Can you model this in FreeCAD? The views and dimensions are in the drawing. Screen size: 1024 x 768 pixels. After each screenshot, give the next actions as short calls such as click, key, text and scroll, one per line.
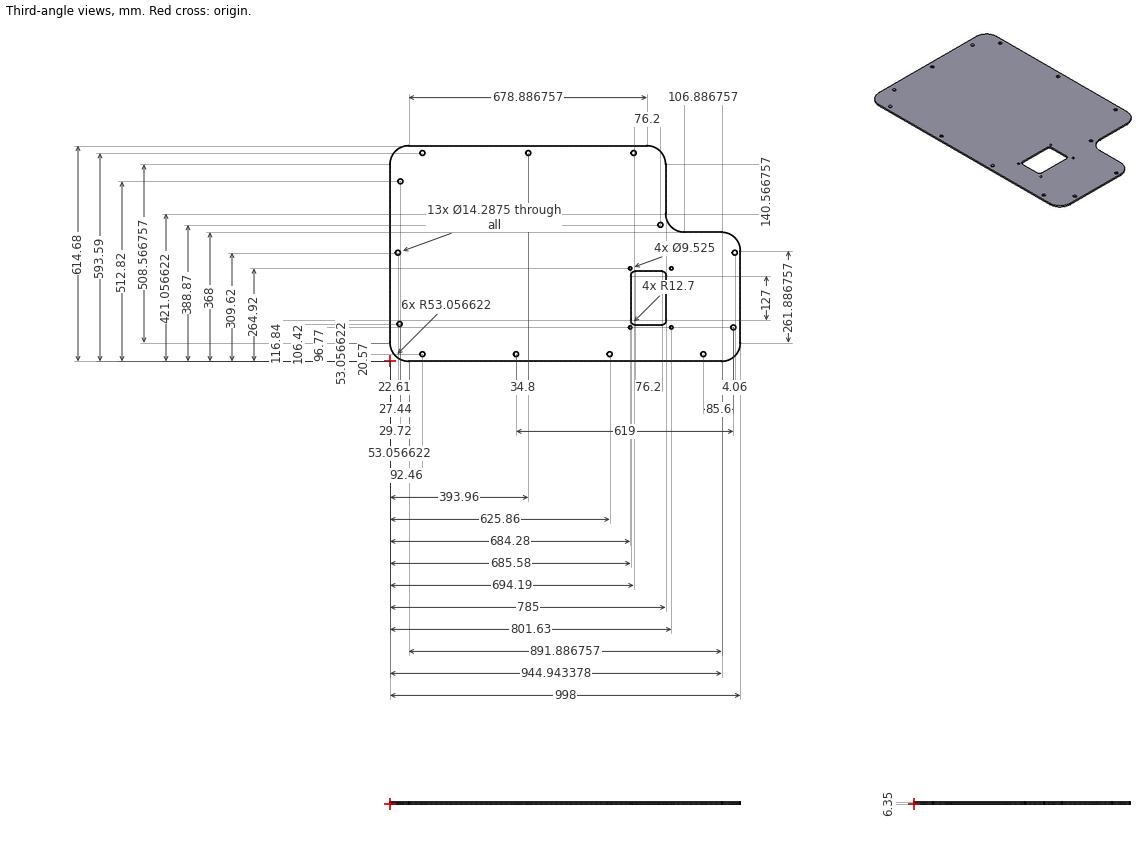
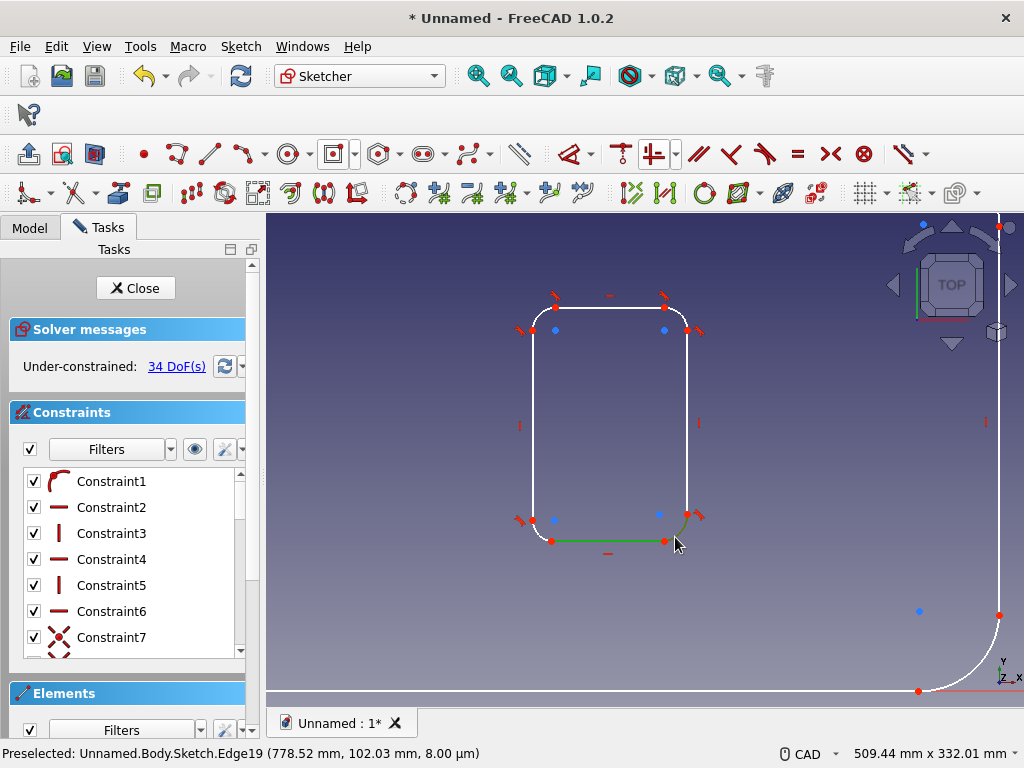
click(765, 154)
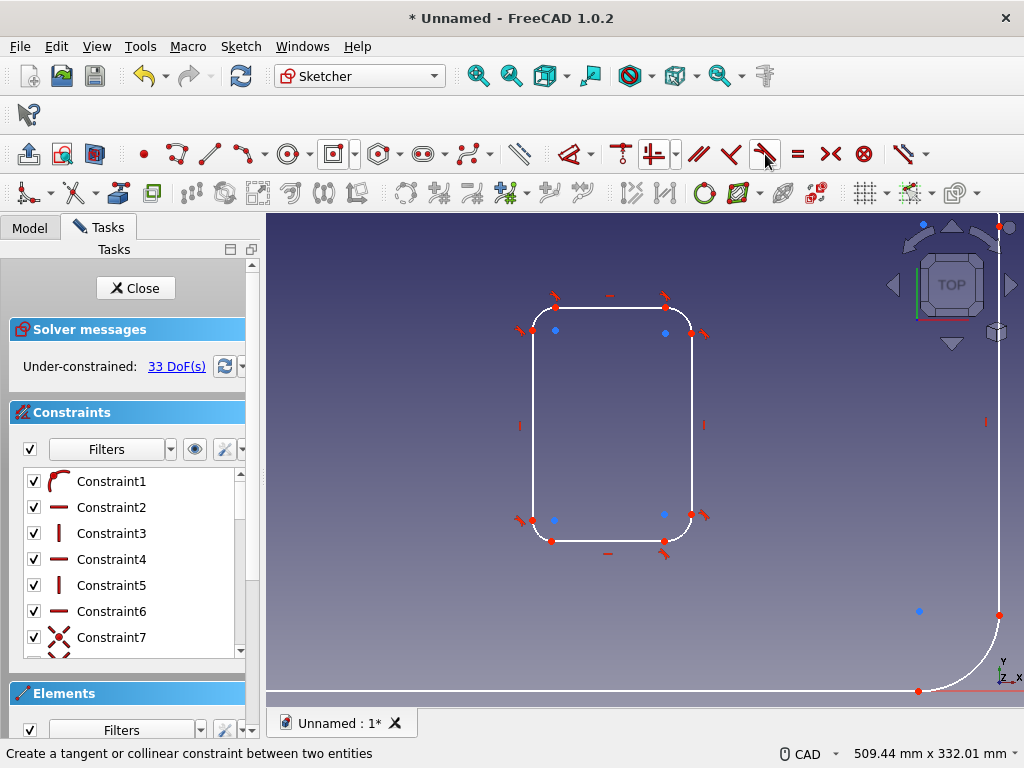
click(631, 541)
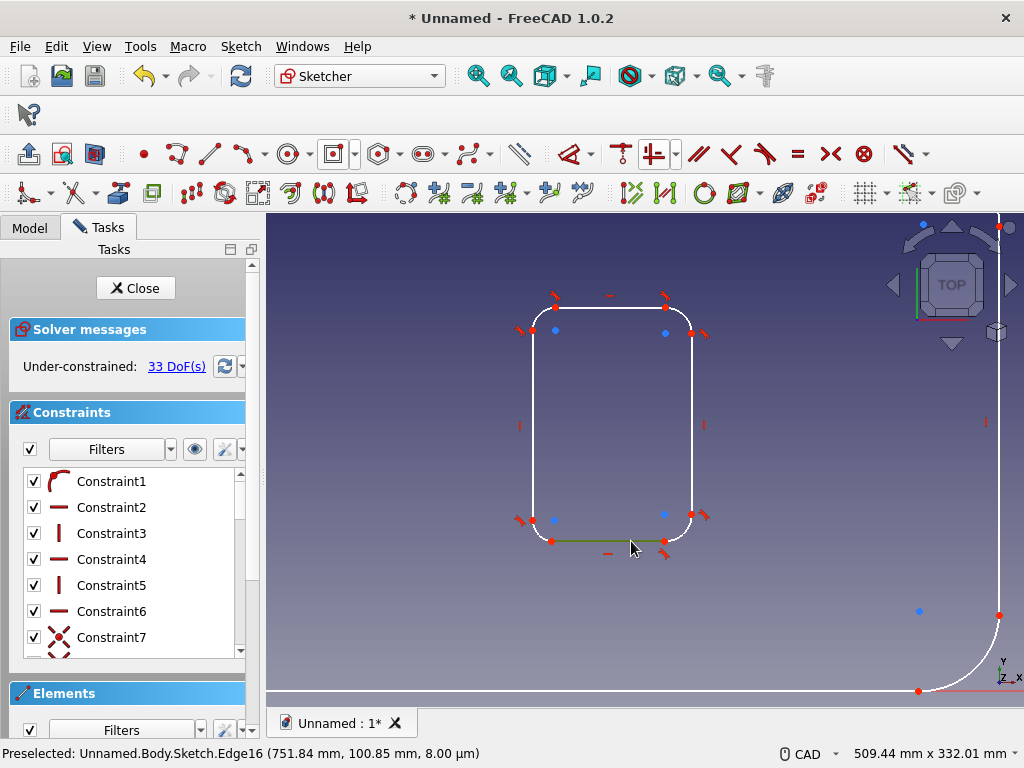
scroll(535, 529, up, 3)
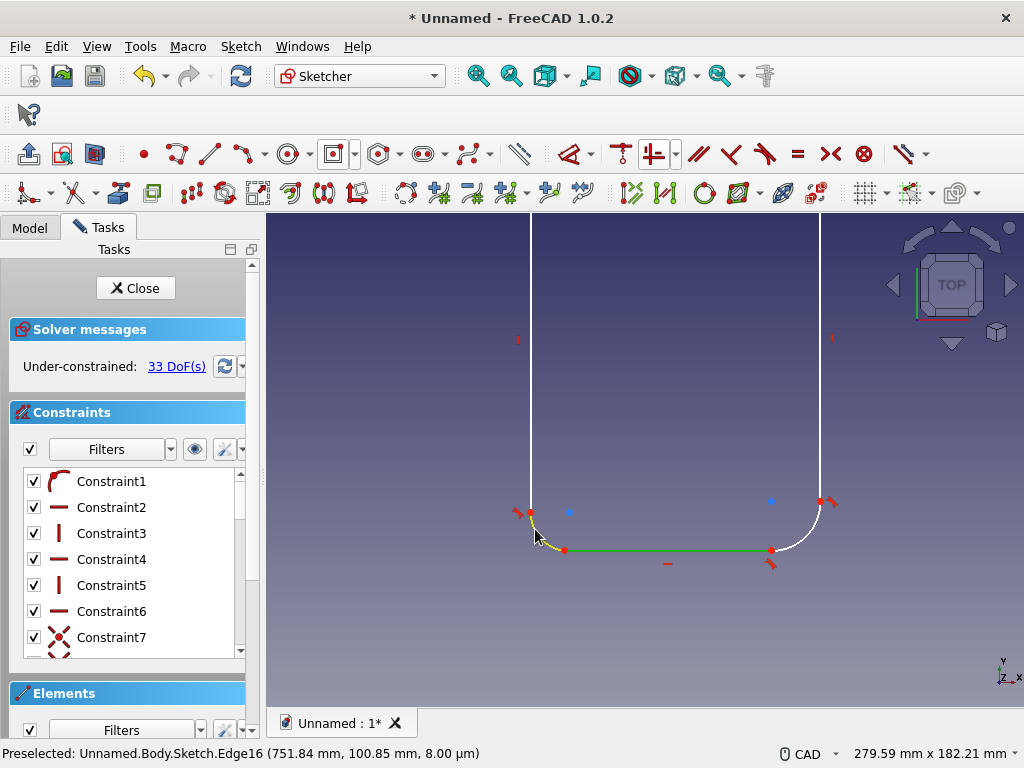
click(534, 529)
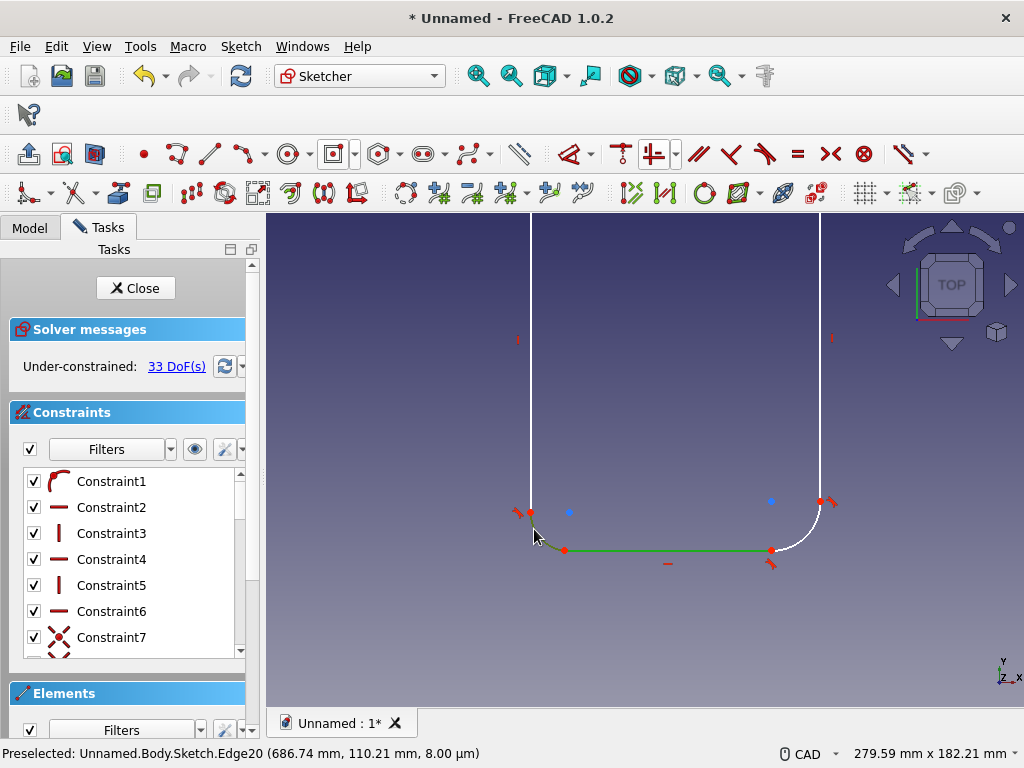
click(765, 154)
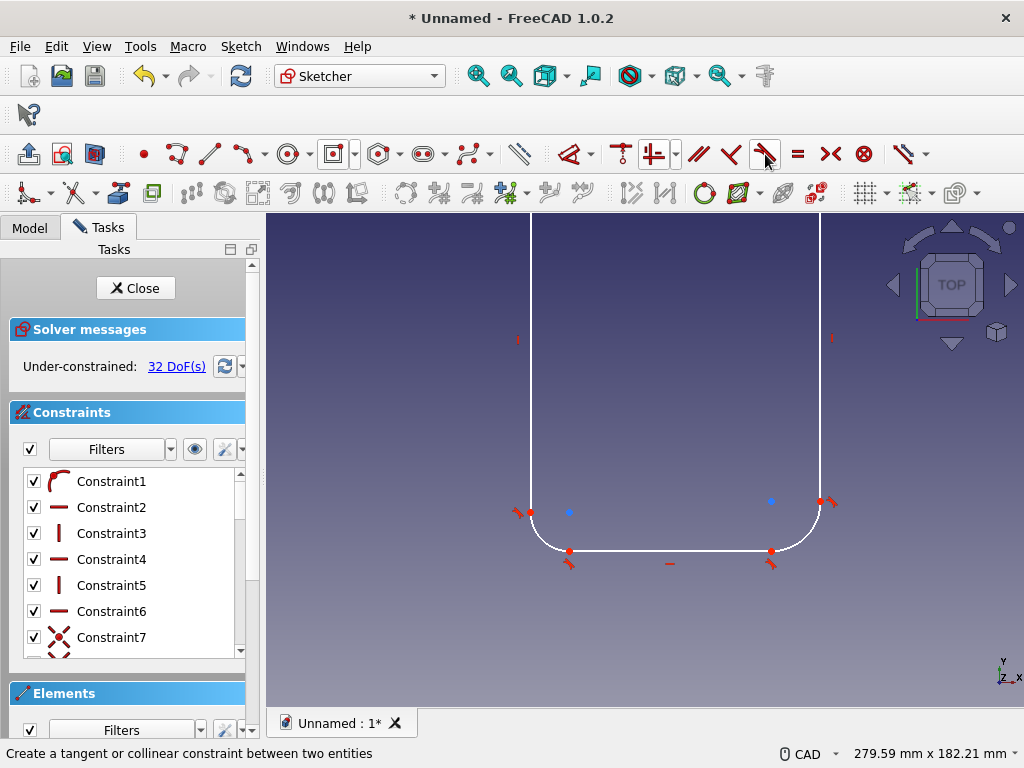
scroll(663, 533, down, 10)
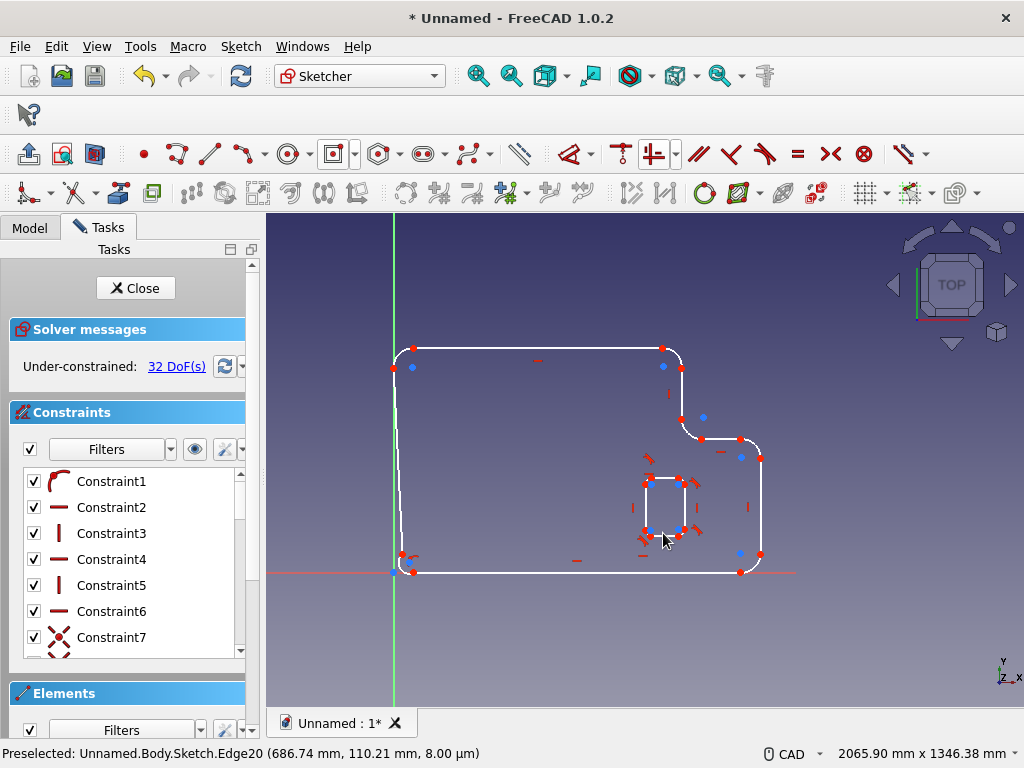
scroll(396, 424, up, 9)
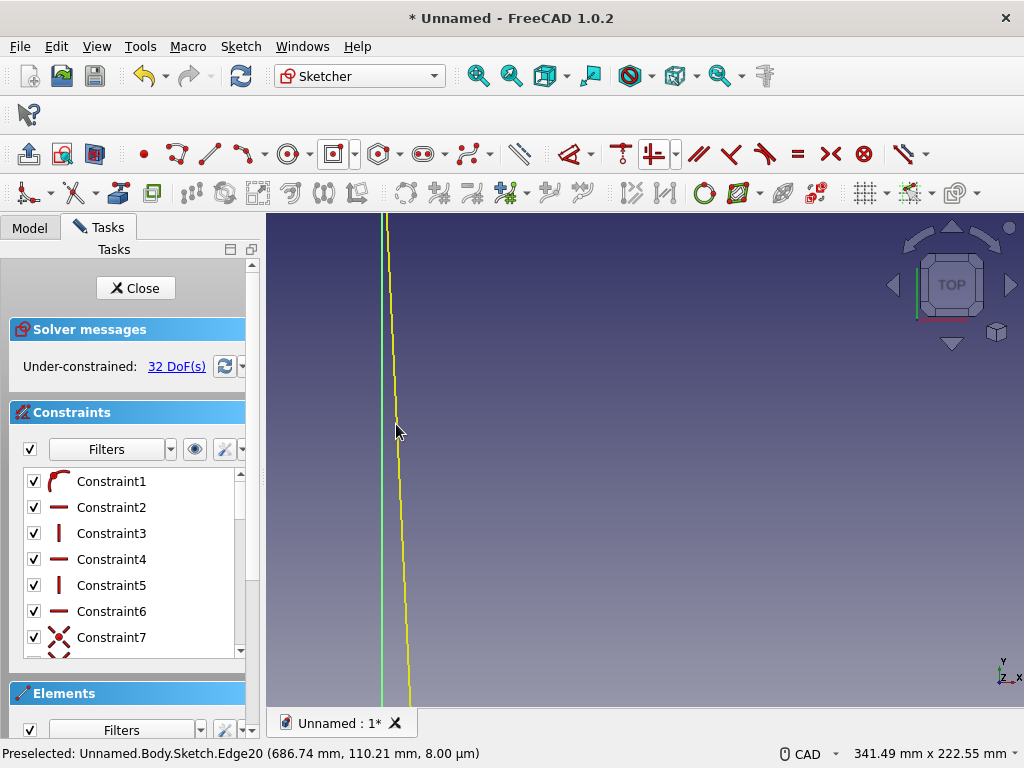
click(397, 423)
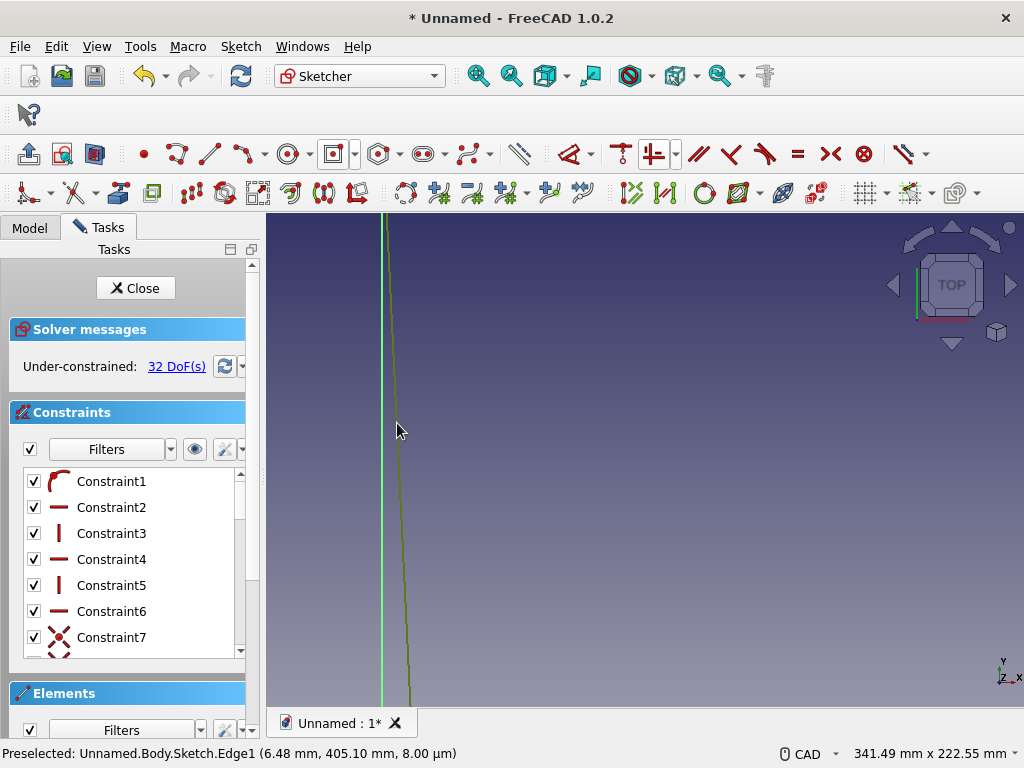
key(v)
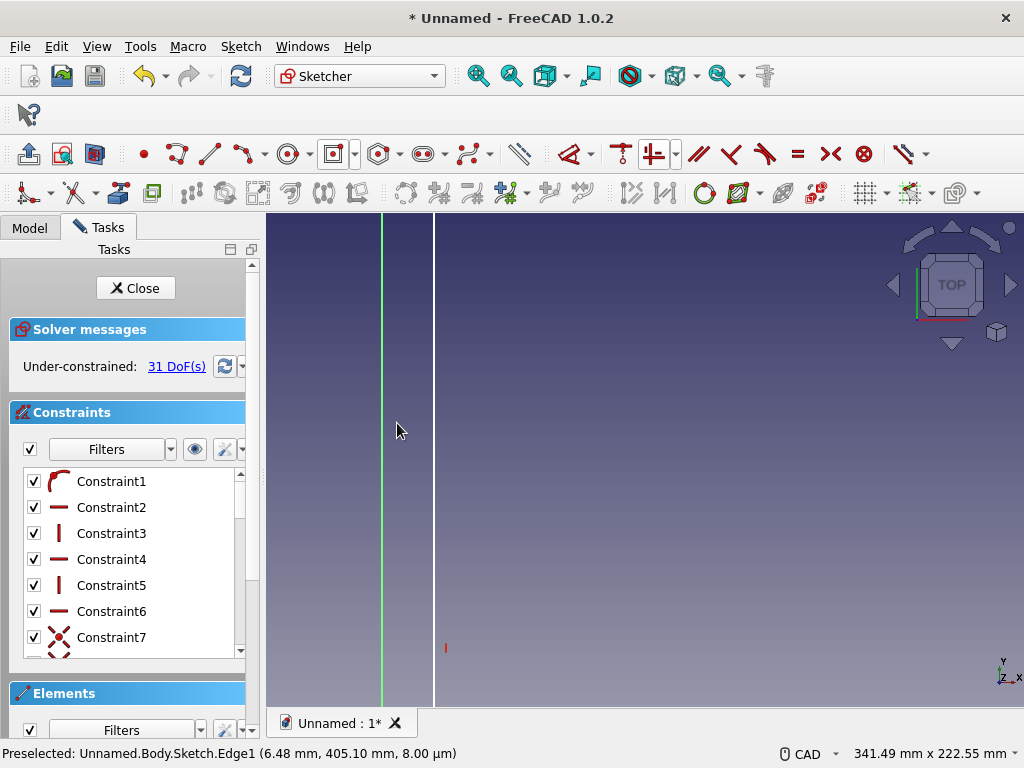
scroll(396, 424, down, 9)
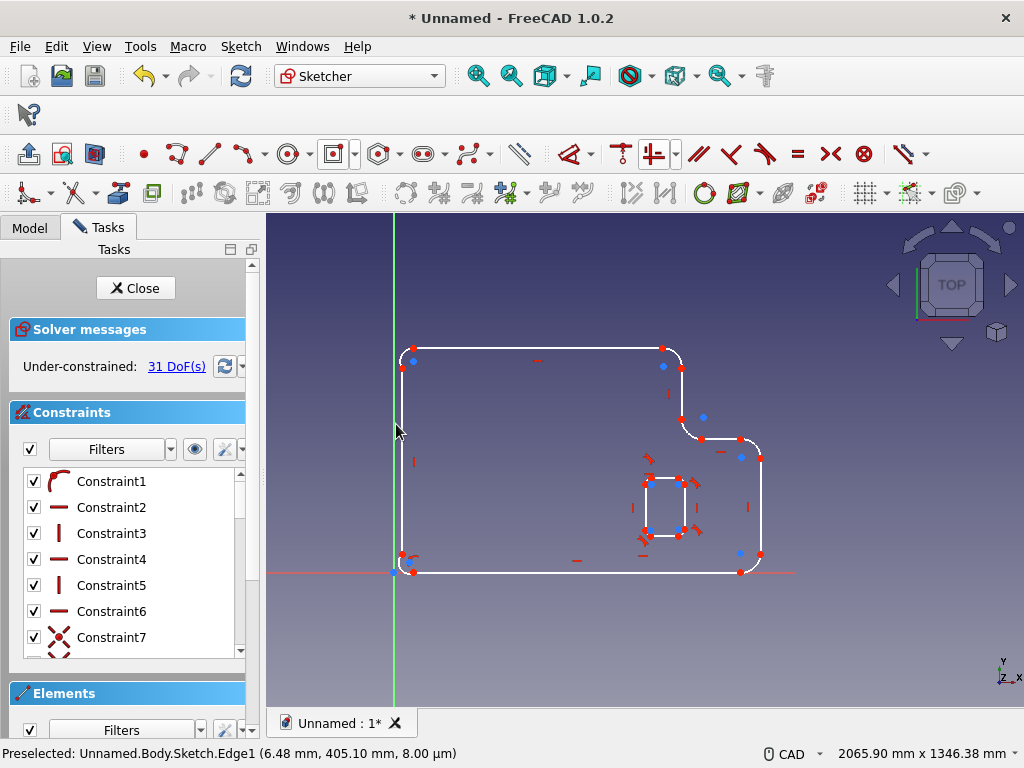
scroll(399, 562, up, 6)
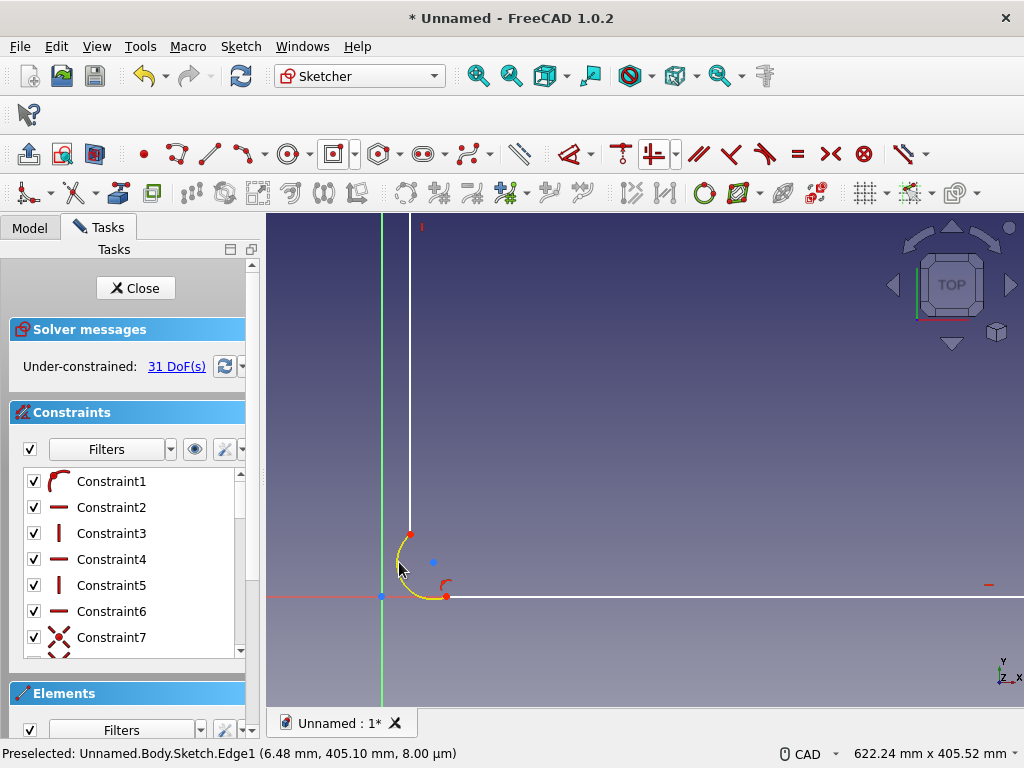
click(397, 562)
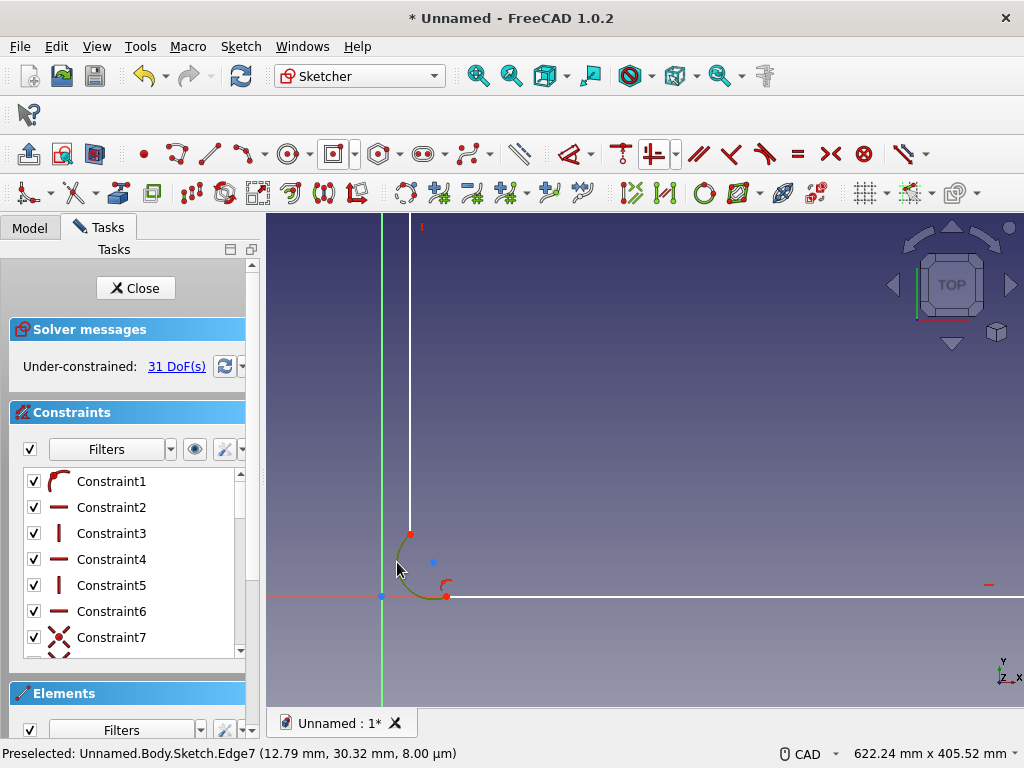
scroll(398, 562, down, 6)